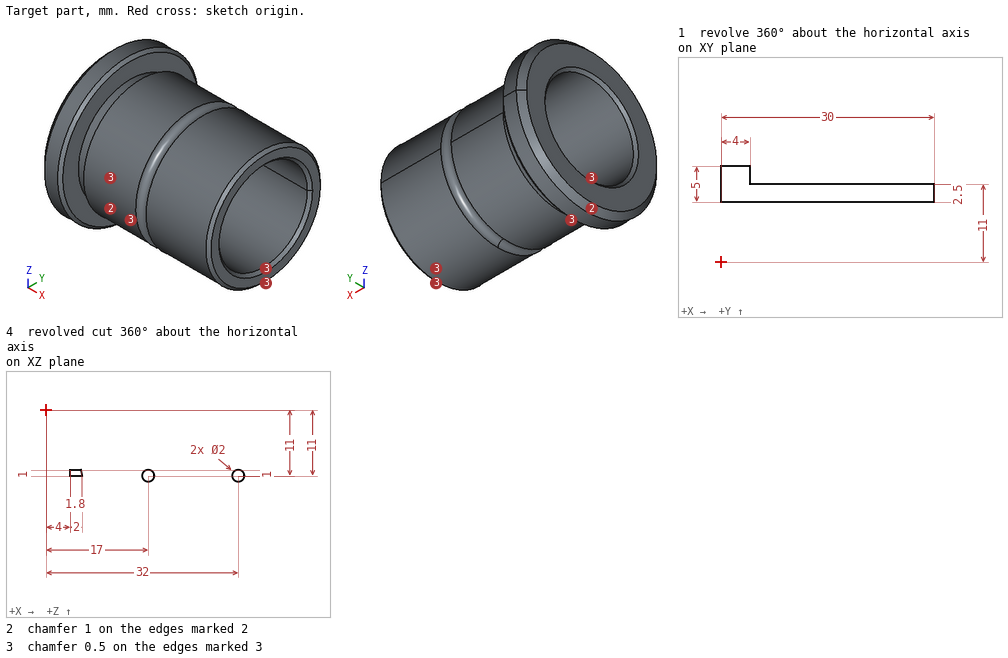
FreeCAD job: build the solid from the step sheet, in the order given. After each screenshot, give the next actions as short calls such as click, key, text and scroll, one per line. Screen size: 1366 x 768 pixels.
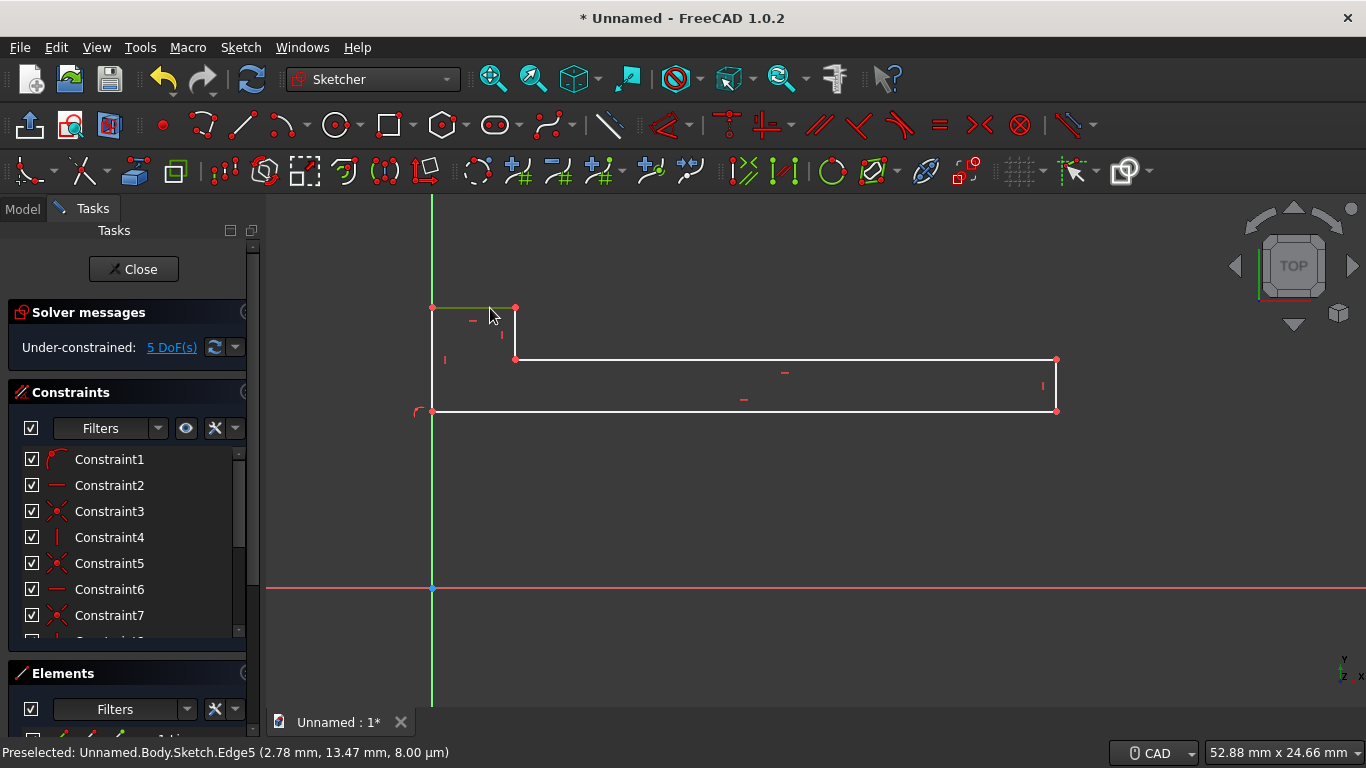
click(692, 126)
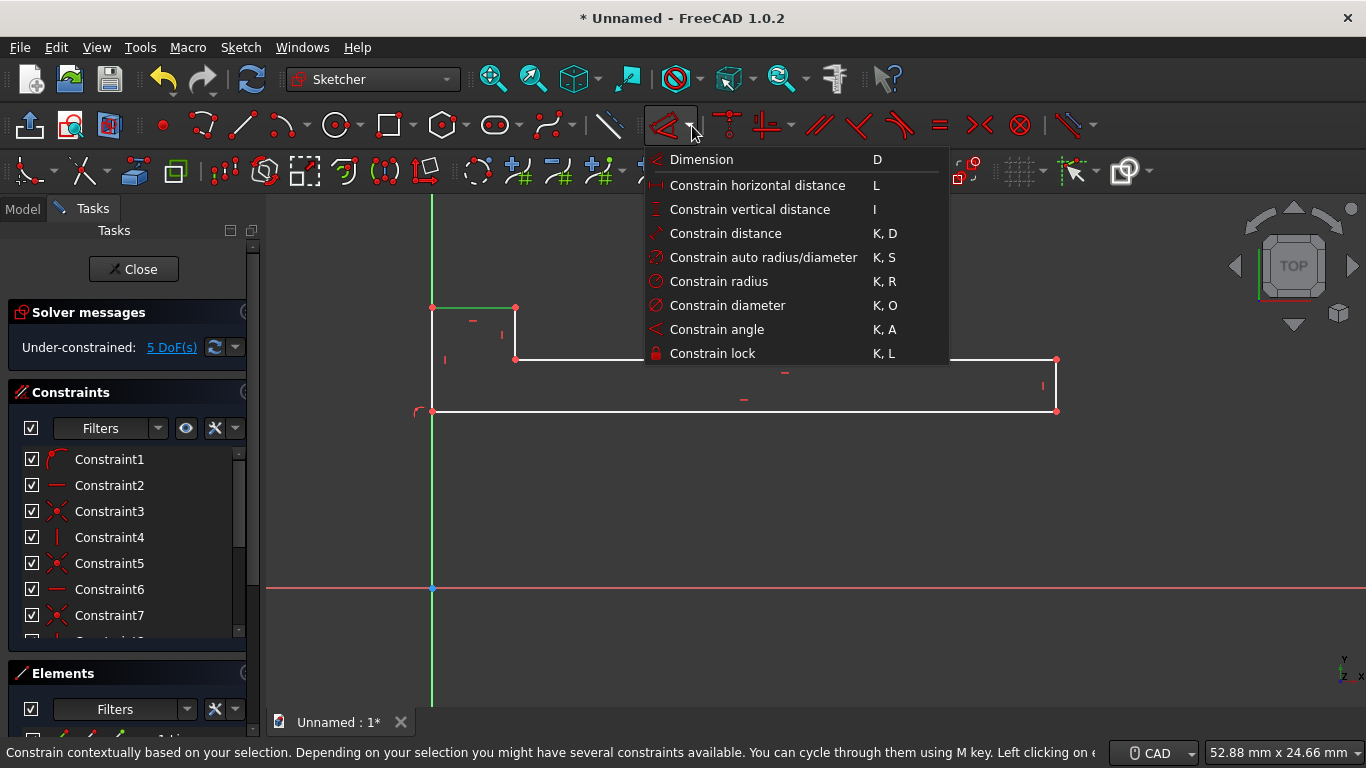
click(797, 185)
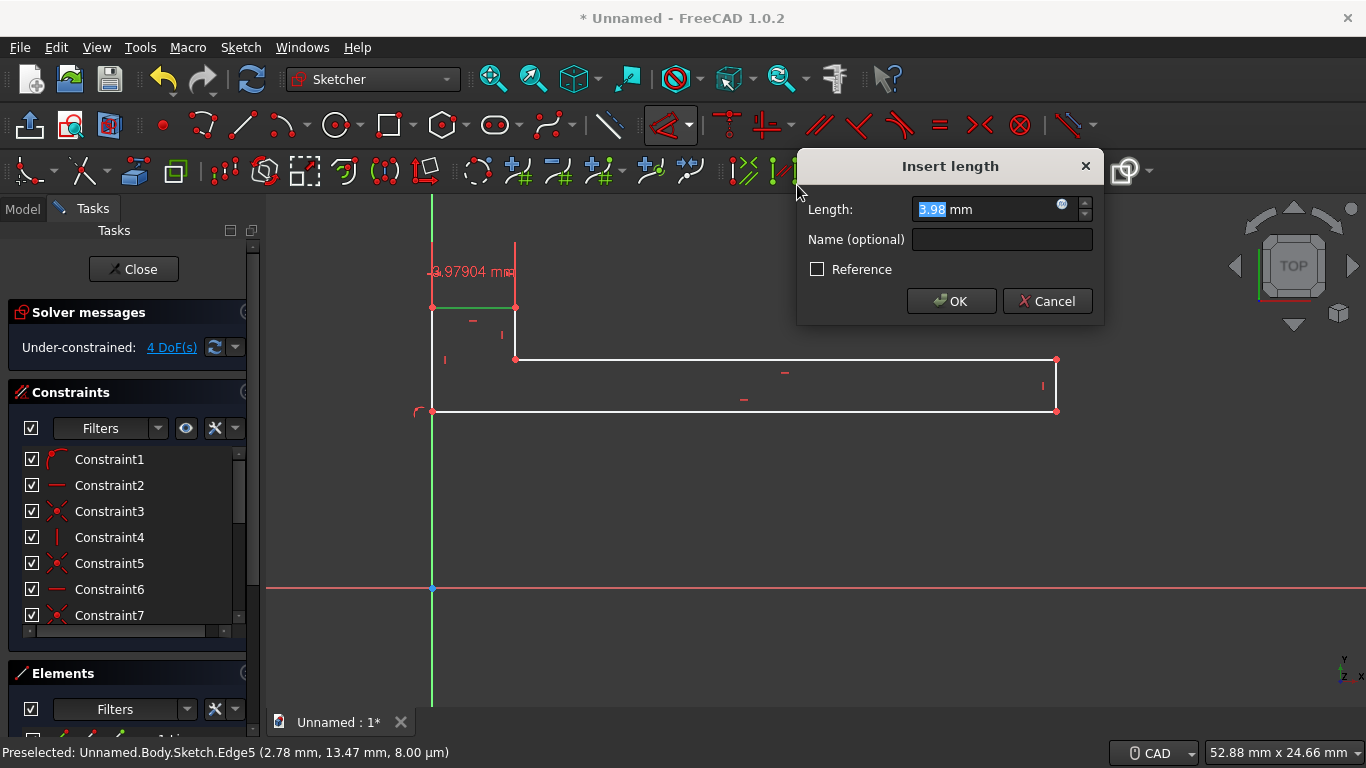
text(4)
key(Return)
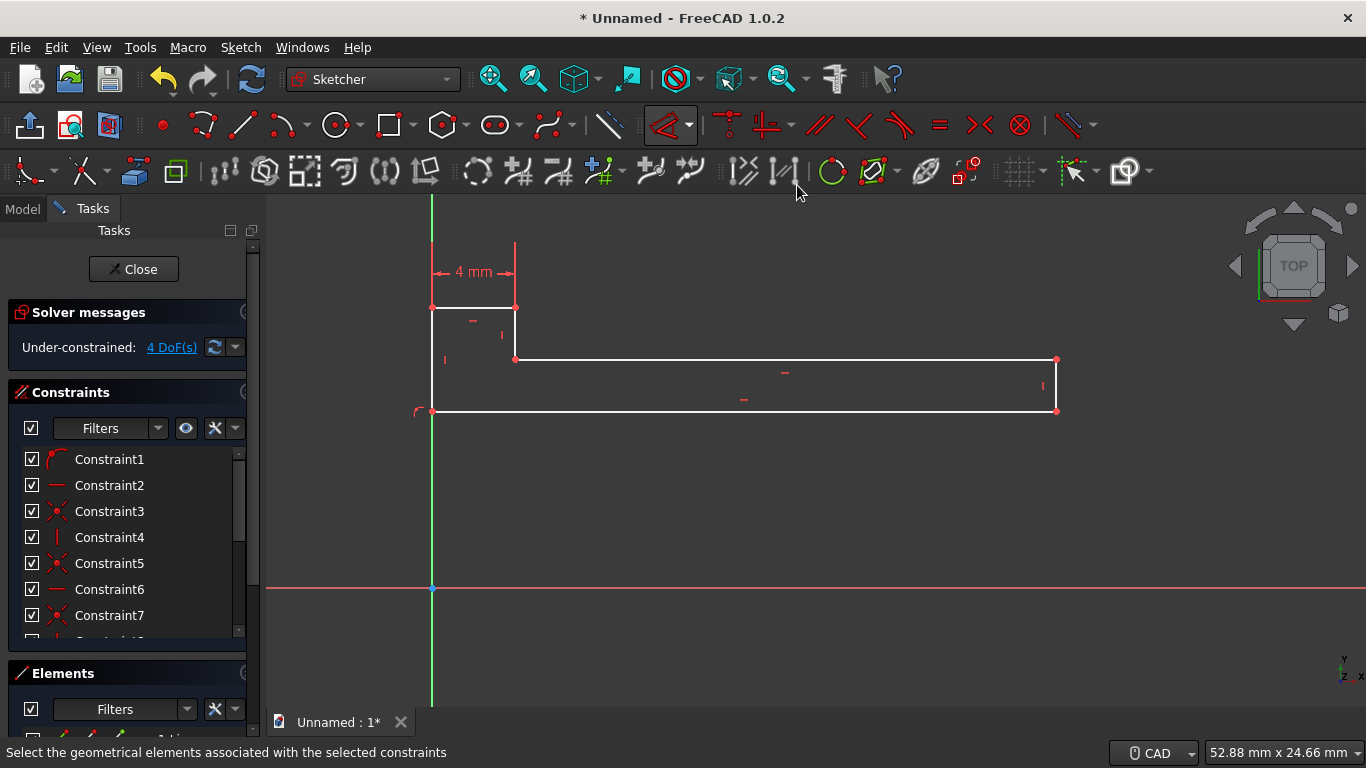
click(432, 339)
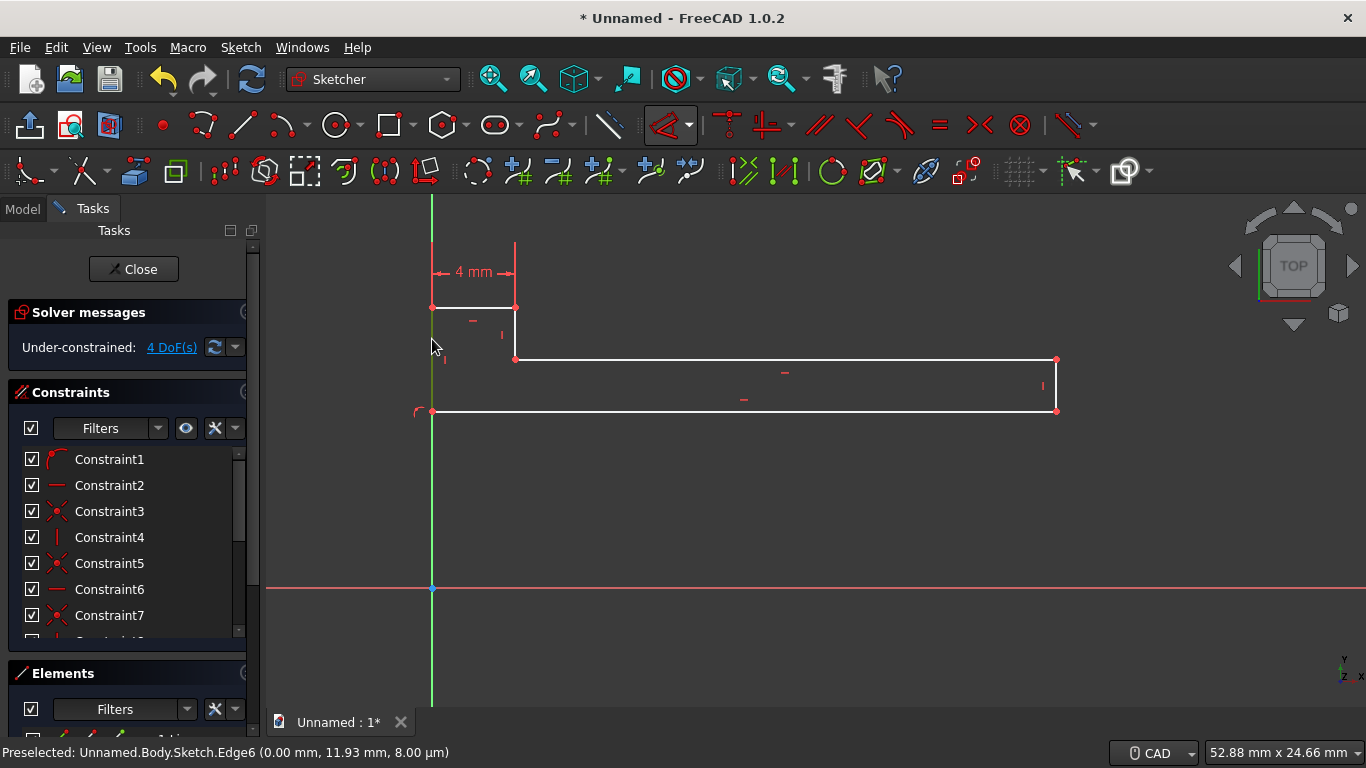
click(692, 126)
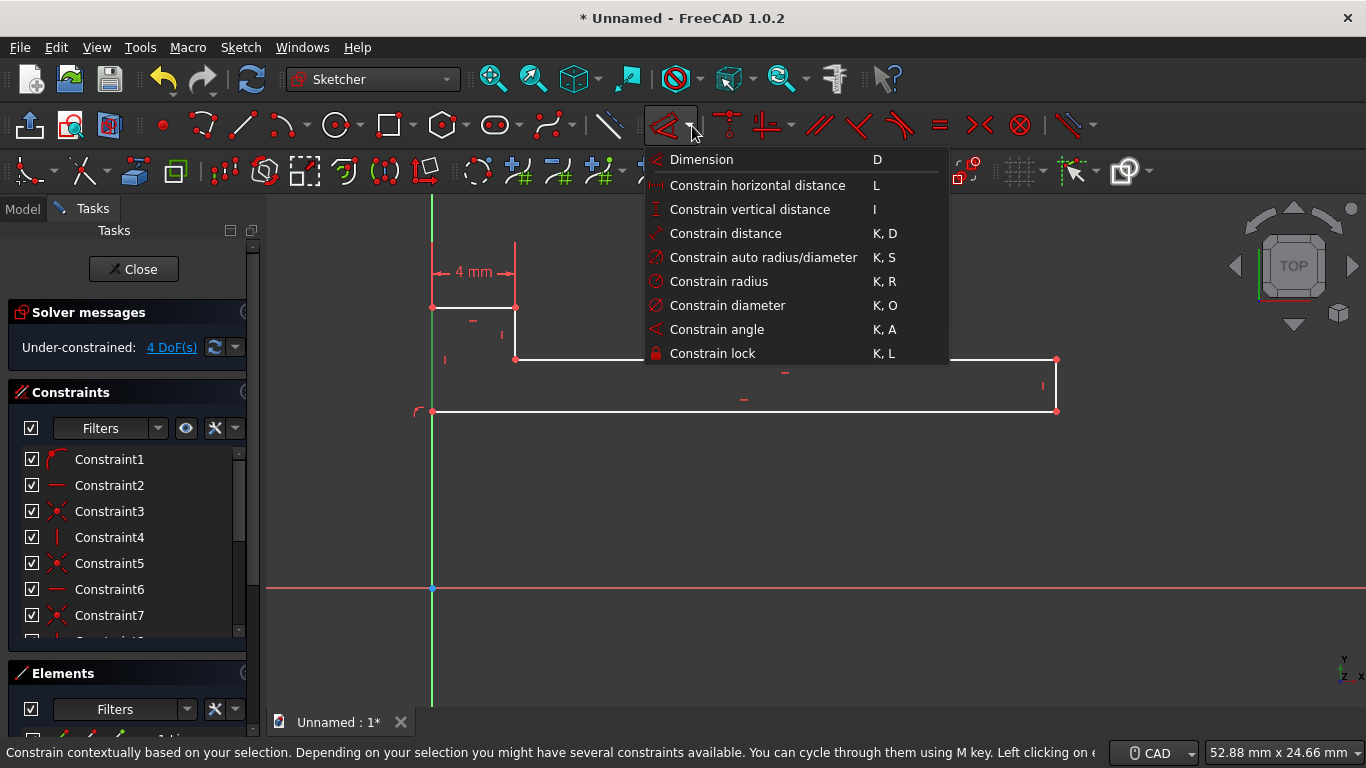
click(797, 209)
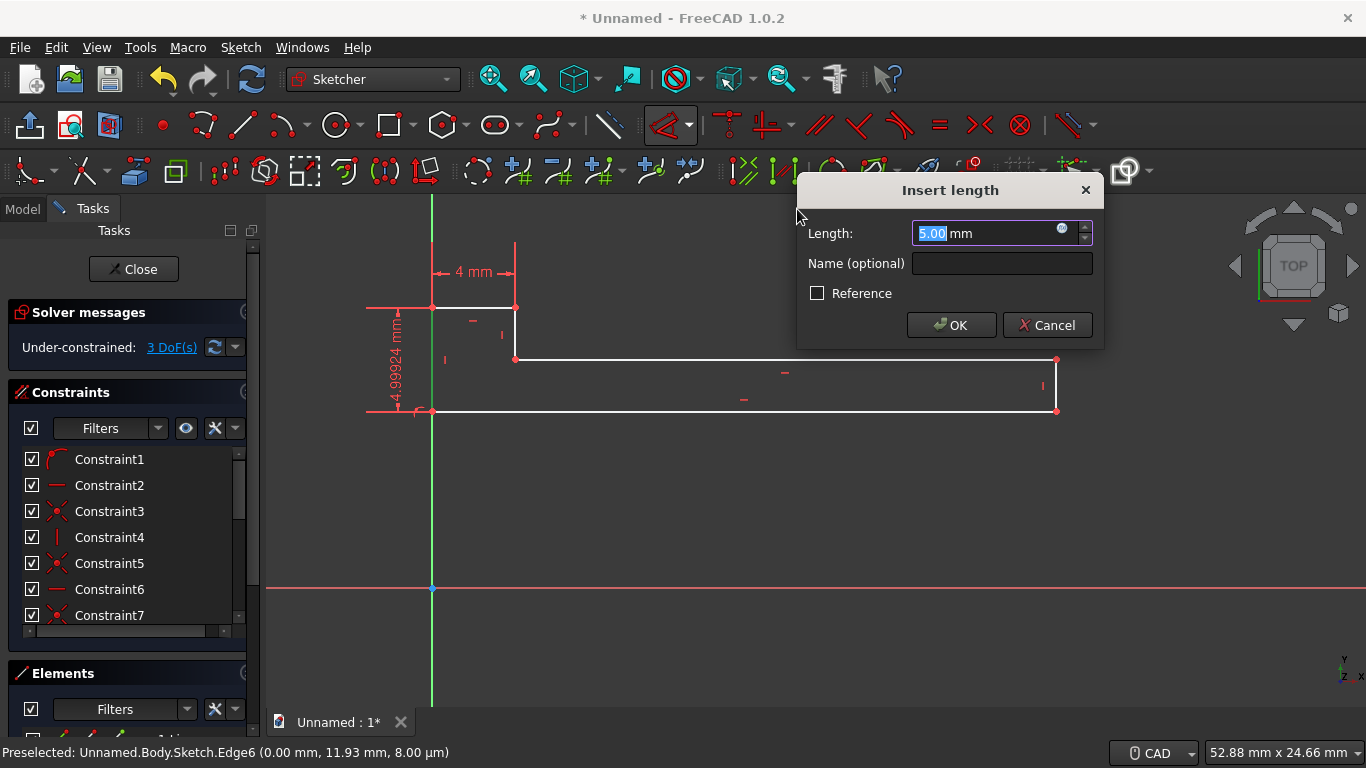
text(5)
key(Return)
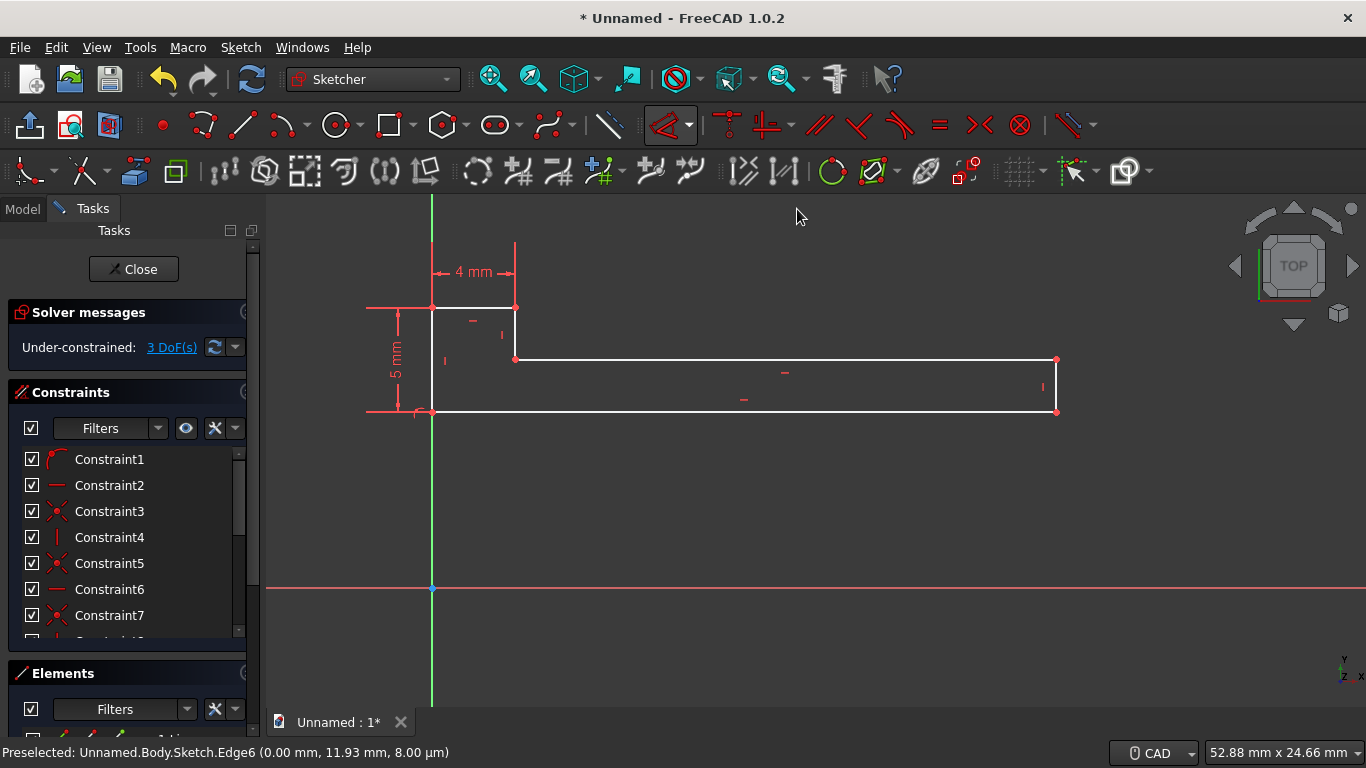
click(619, 412)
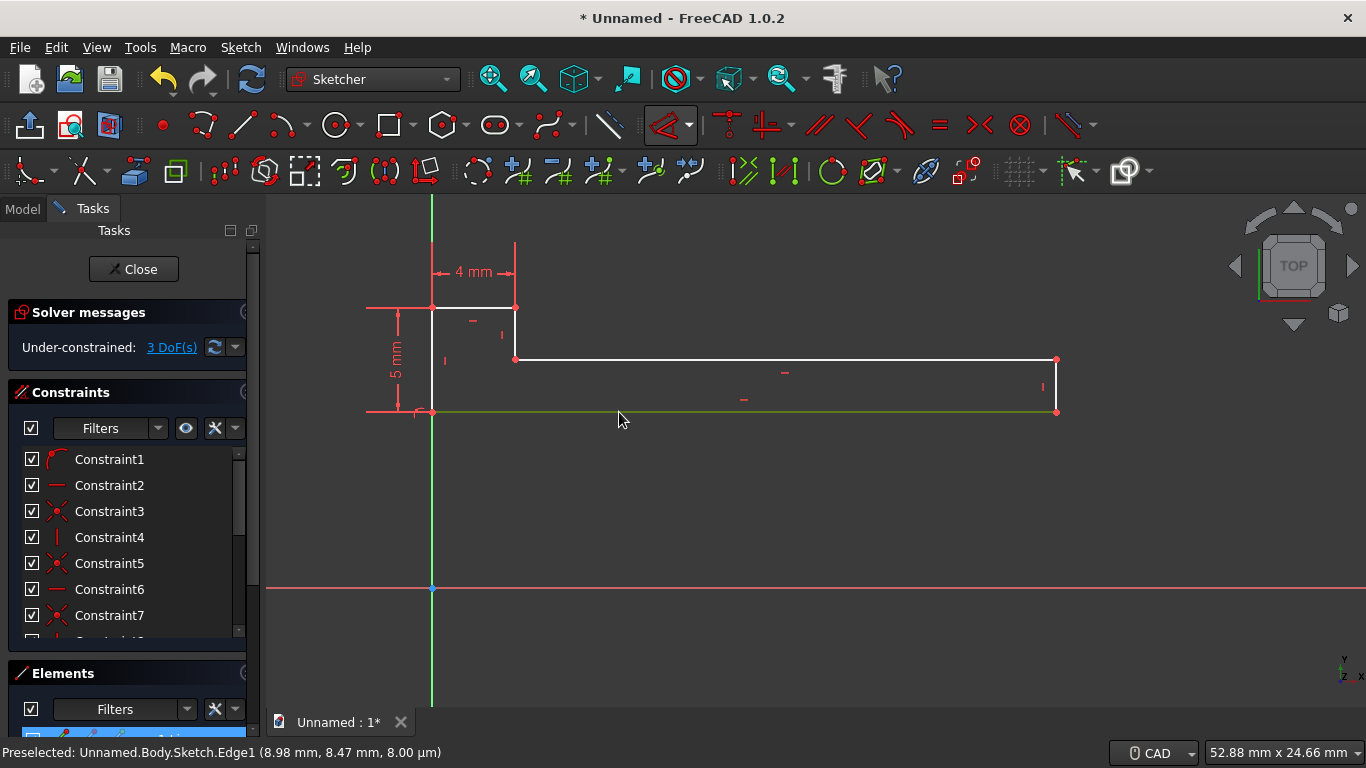
key(l)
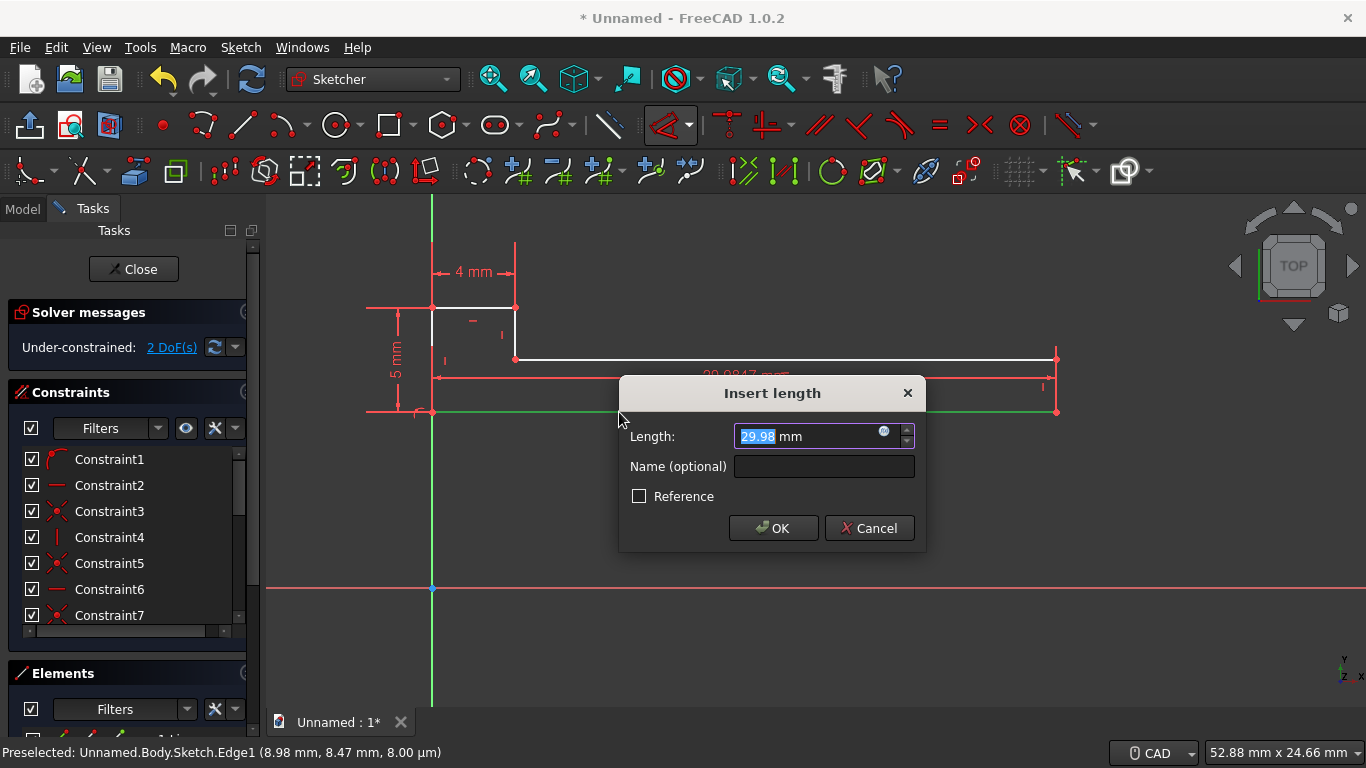
text(30)
key(Return)